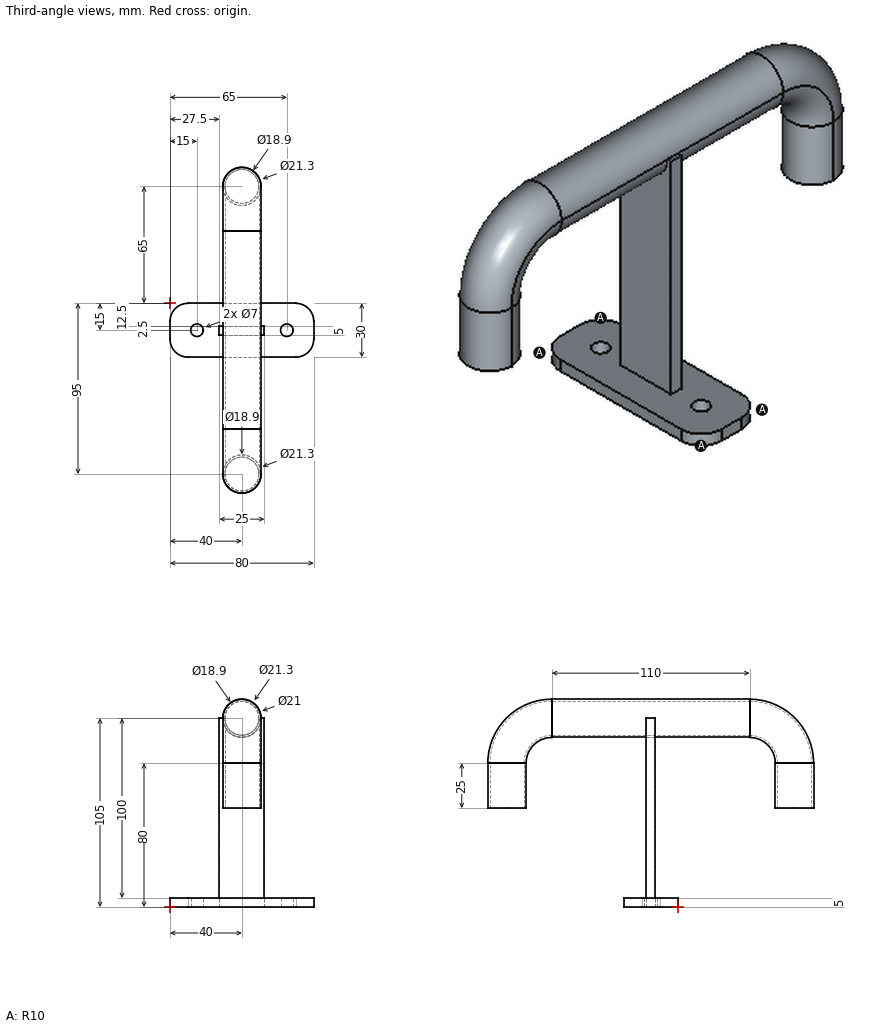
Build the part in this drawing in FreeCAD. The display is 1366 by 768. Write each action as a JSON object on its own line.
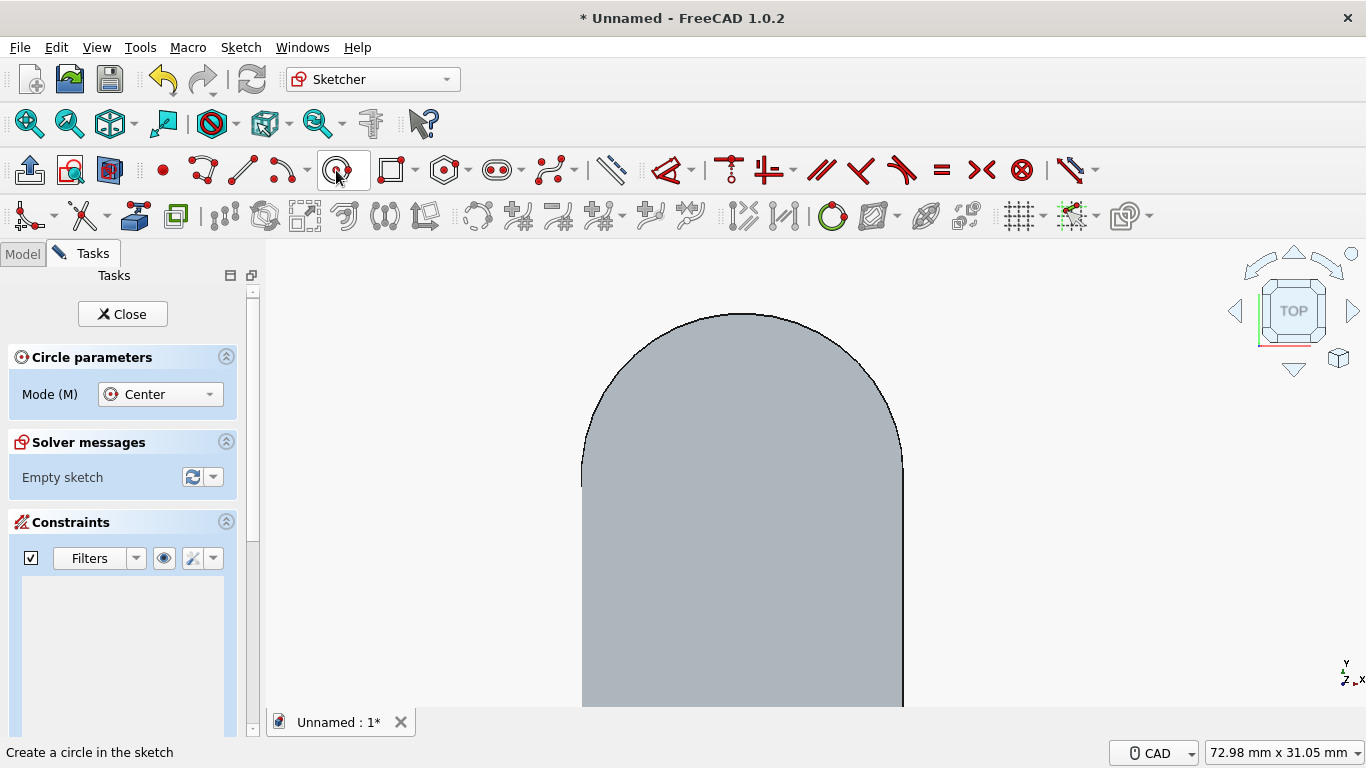
{"action": "left_click", "coordinate": [742, 474]}
{"action": "mouse_move", "coordinate": [856, 361]}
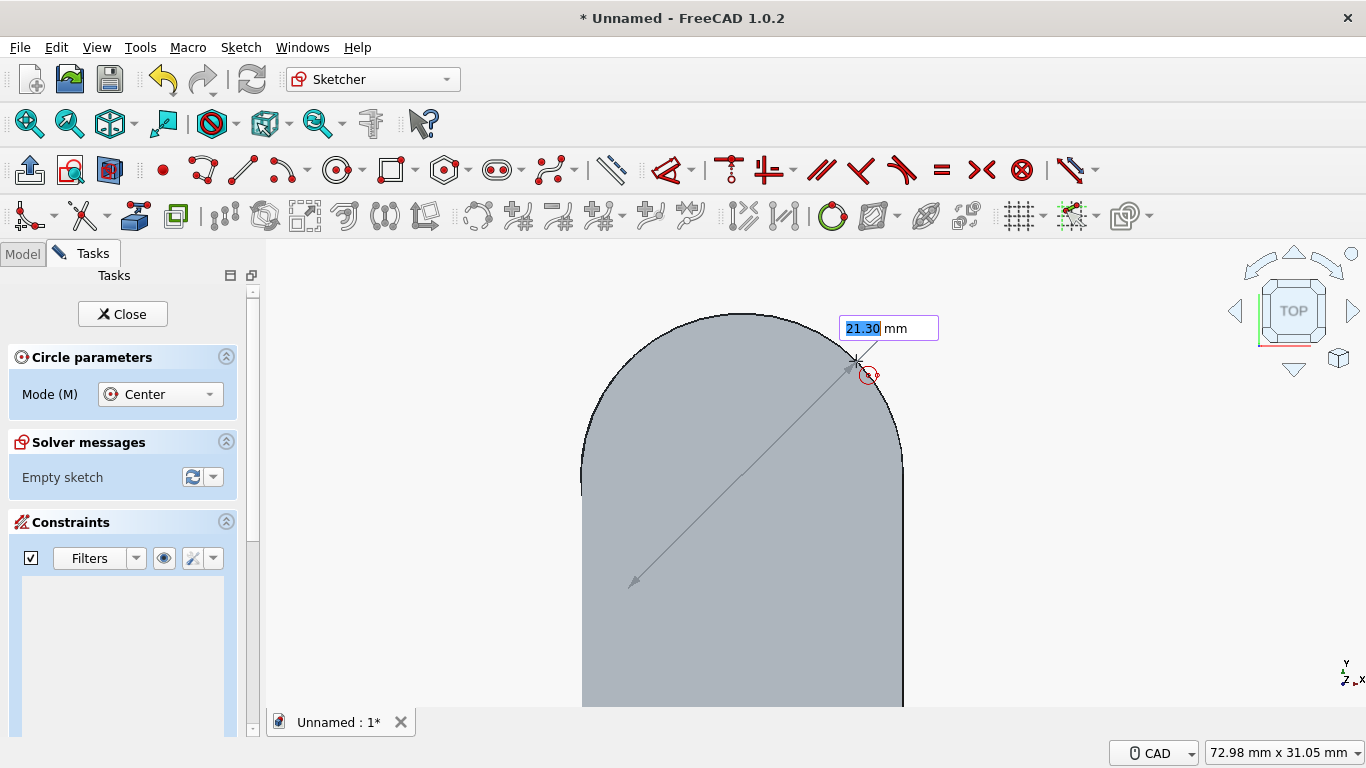
{"action": "type", "text": "21.3"}
{"action": "key", "text": "Return"}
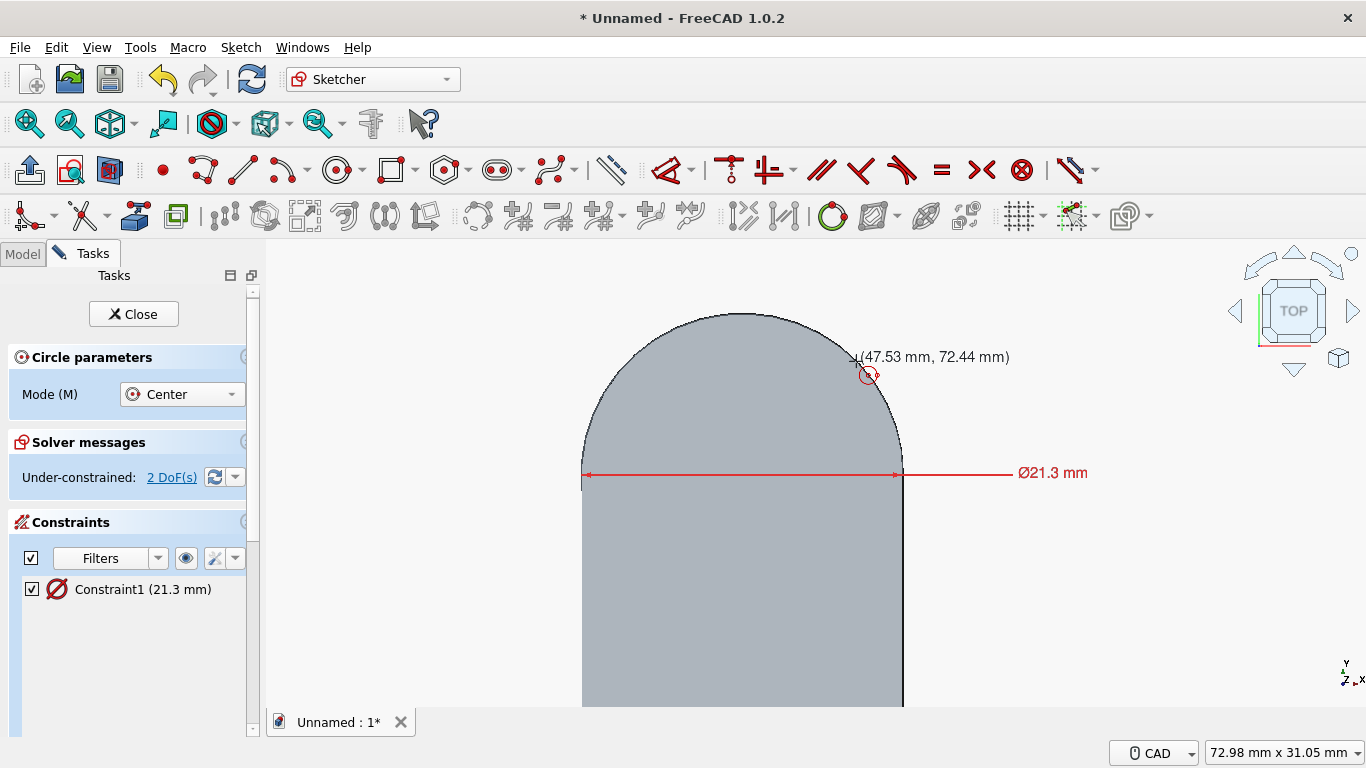
{"action": "left_click", "coordinate": [742, 475]}
{"action": "mouse_move", "coordinate": [843, 373]}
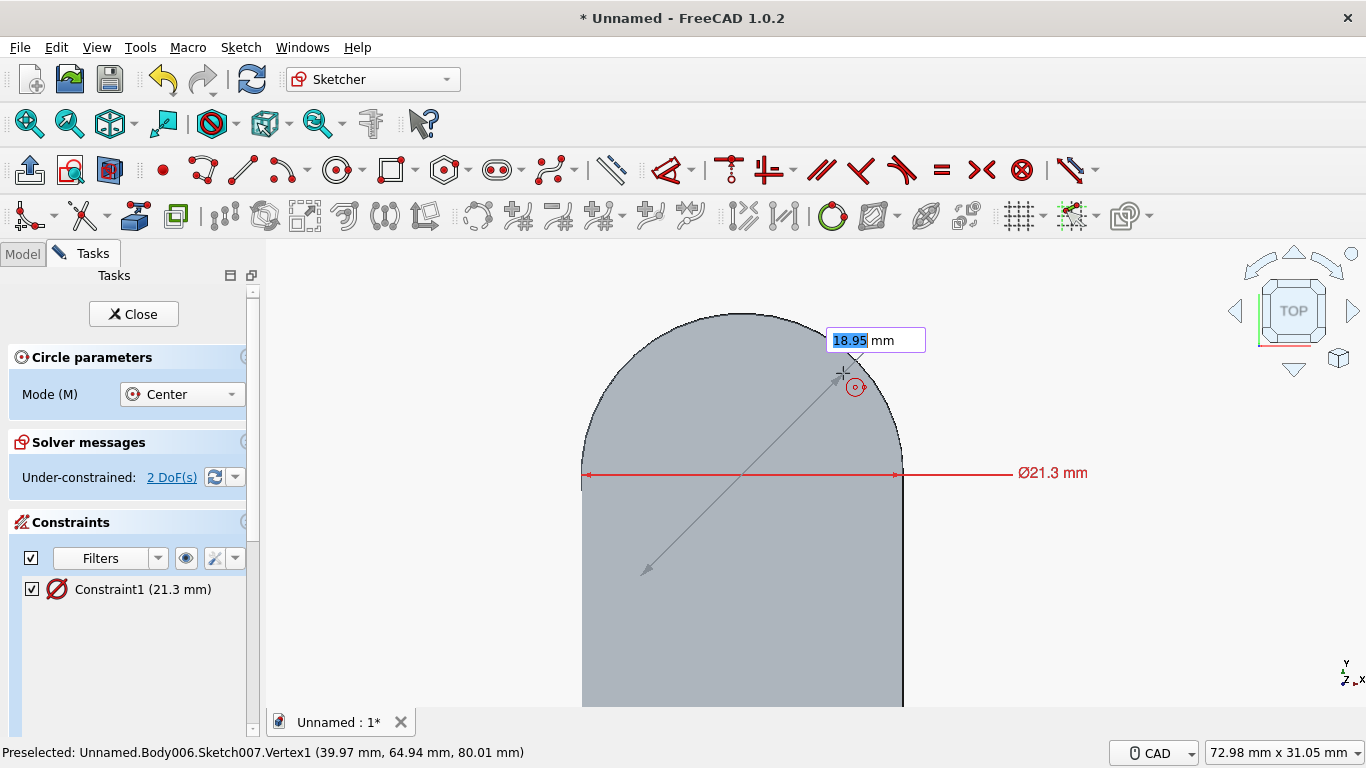
{"action": "type", "text": "18.9"}
{"action": "key", "text": "Return"}
{"action": "key", "text": "Escape"}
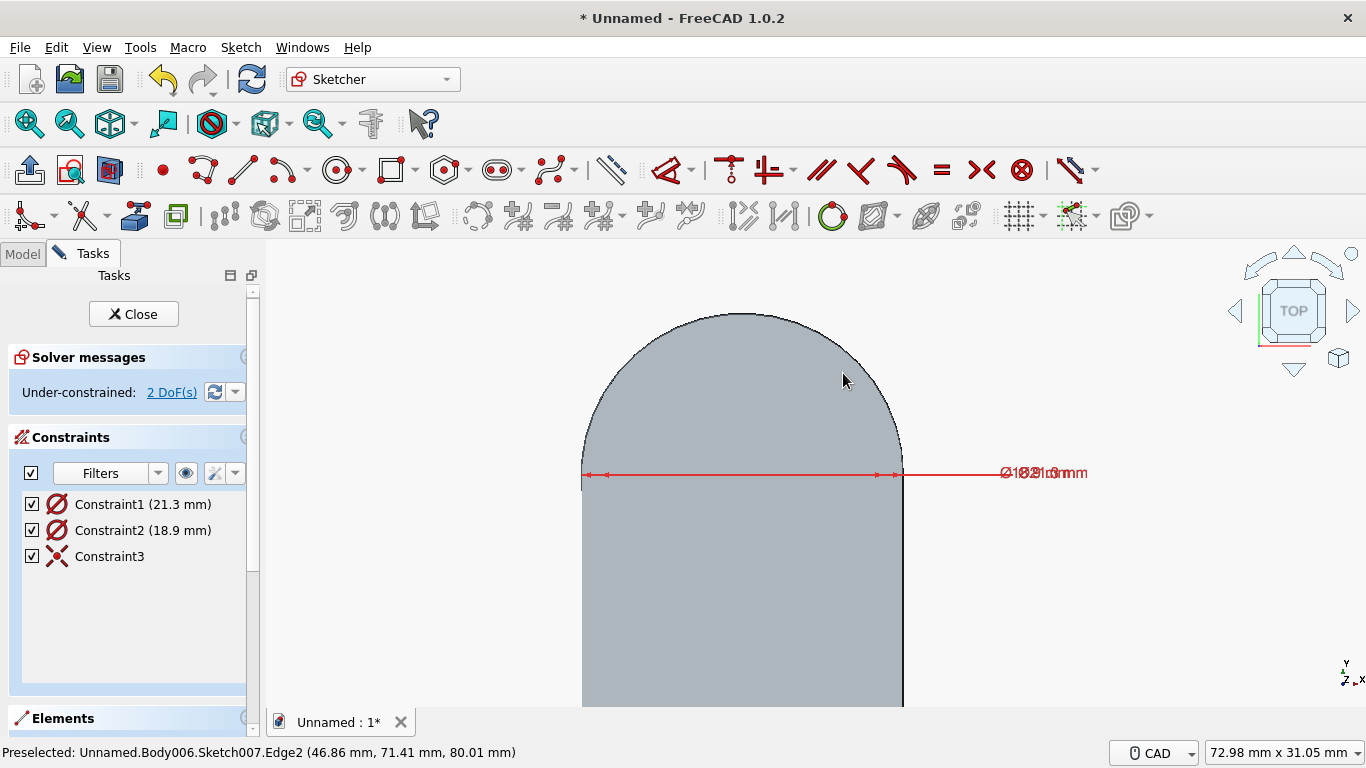
{"action": "left_click", "coordinate": [666, 170]}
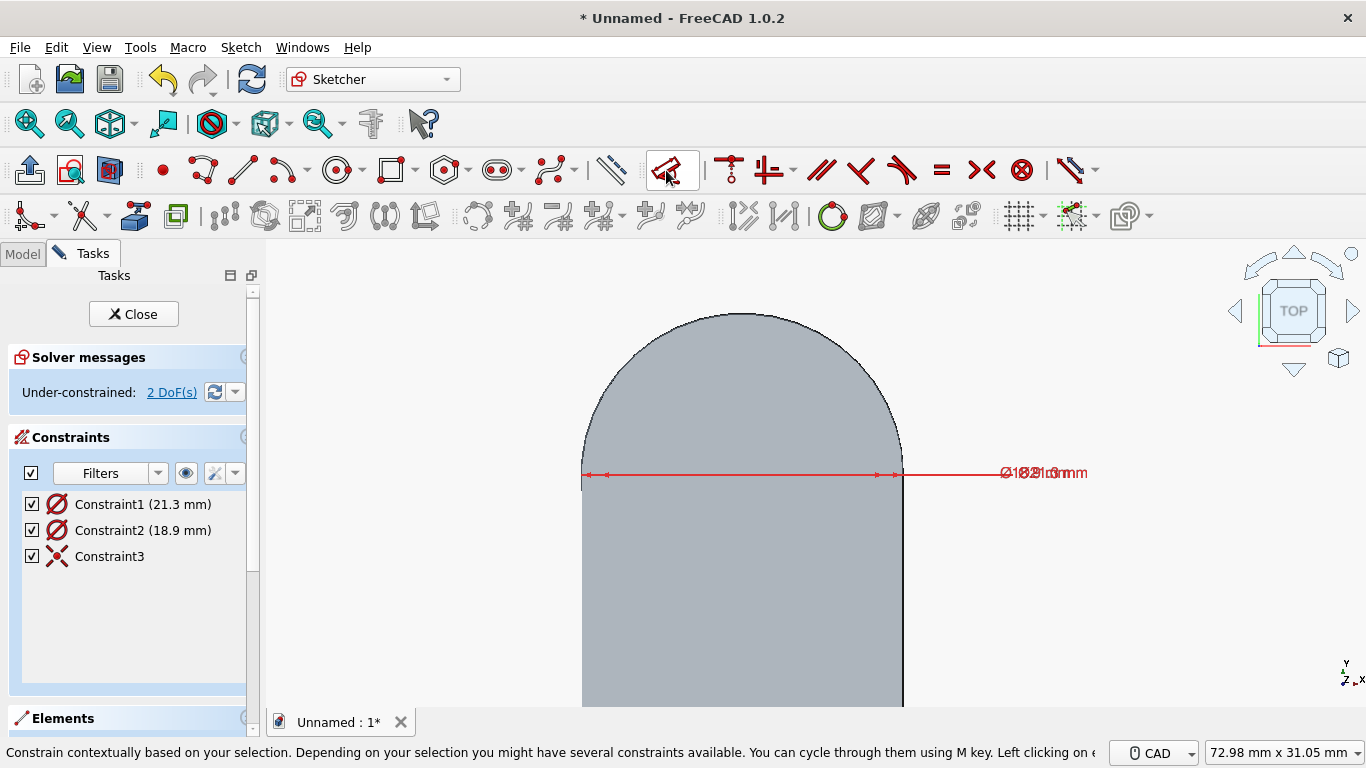
{"action": "left_click", "coordinate": [742, 475]}
{"action": "left_click", "coordinate": [518, 441]}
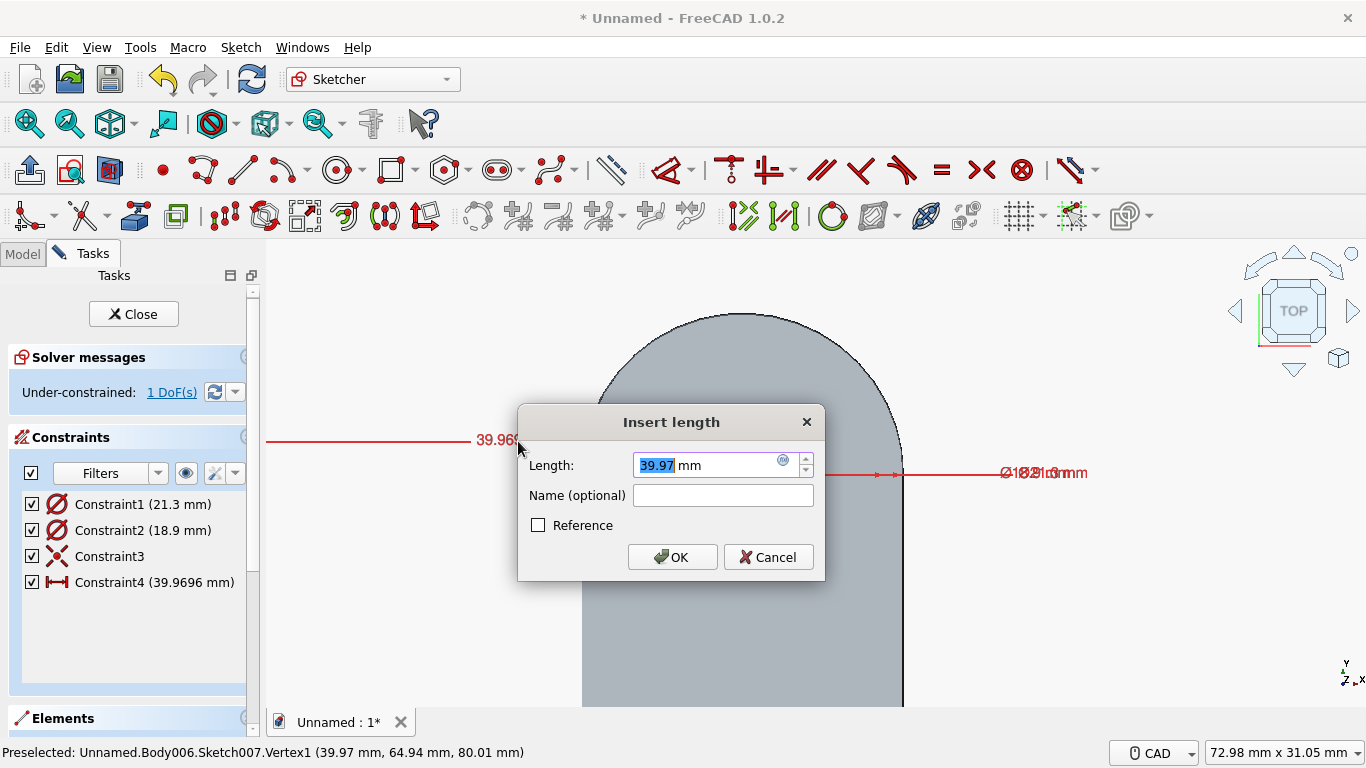
{"action": "type", "text": "40"}
{"action": "key", "text": "Return"}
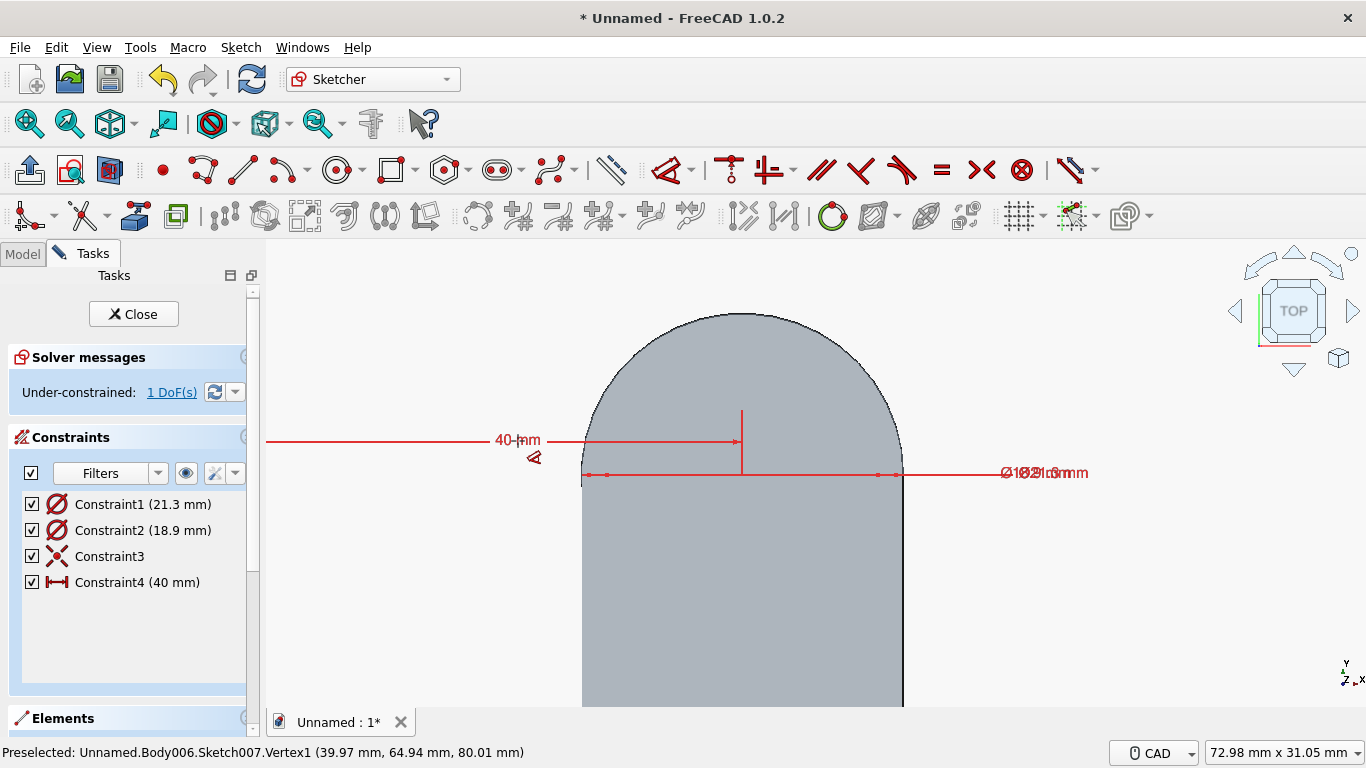
{"action": "left_click", "coordinate": [742, 475]}
{"action": "left_click", "coordinate": [776, 577]}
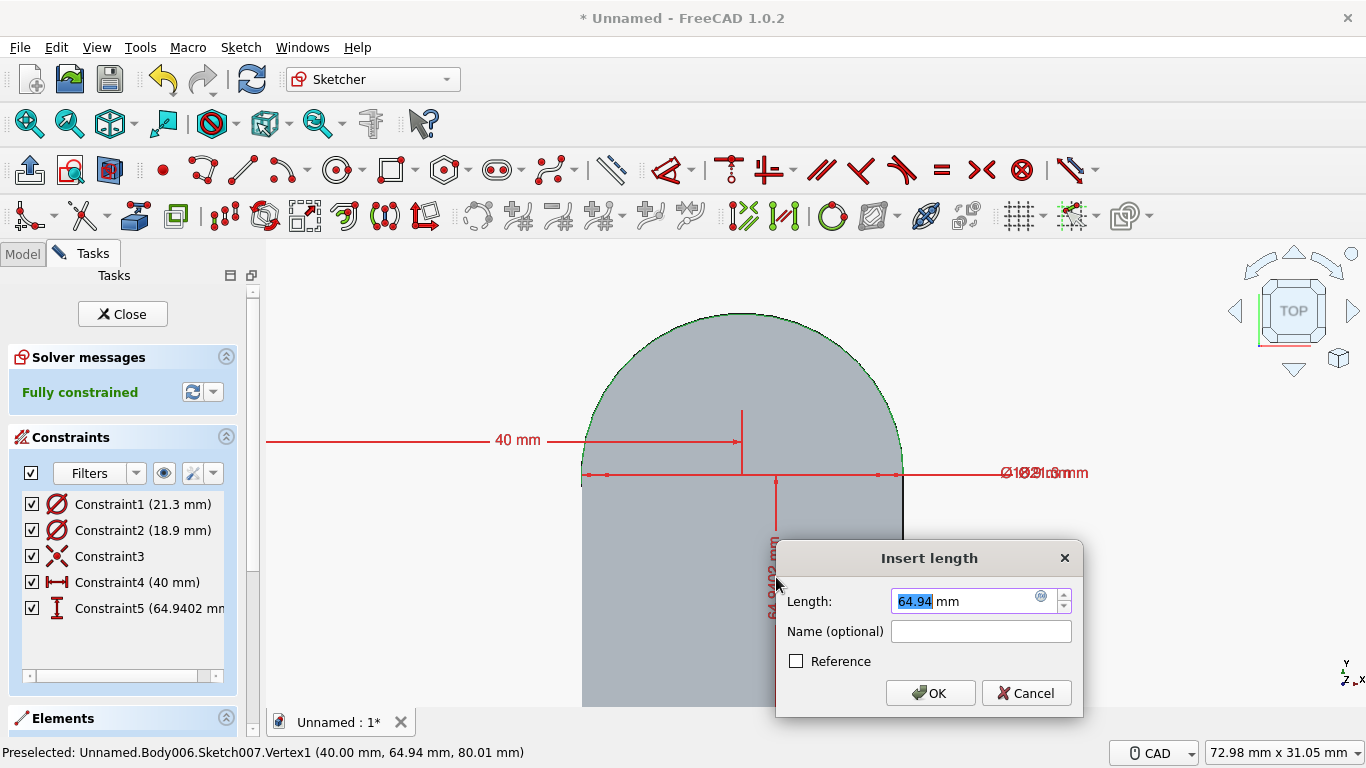
{"action": "type", "text": "65"}
{"action": "key", "text": "Return"}
{"action": "key", "text": "Escape"}